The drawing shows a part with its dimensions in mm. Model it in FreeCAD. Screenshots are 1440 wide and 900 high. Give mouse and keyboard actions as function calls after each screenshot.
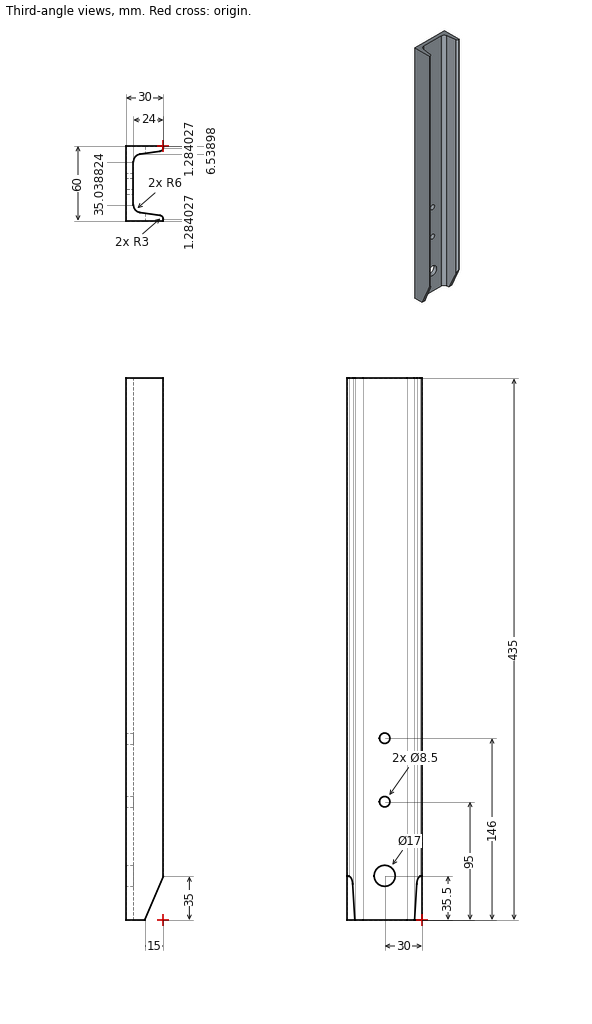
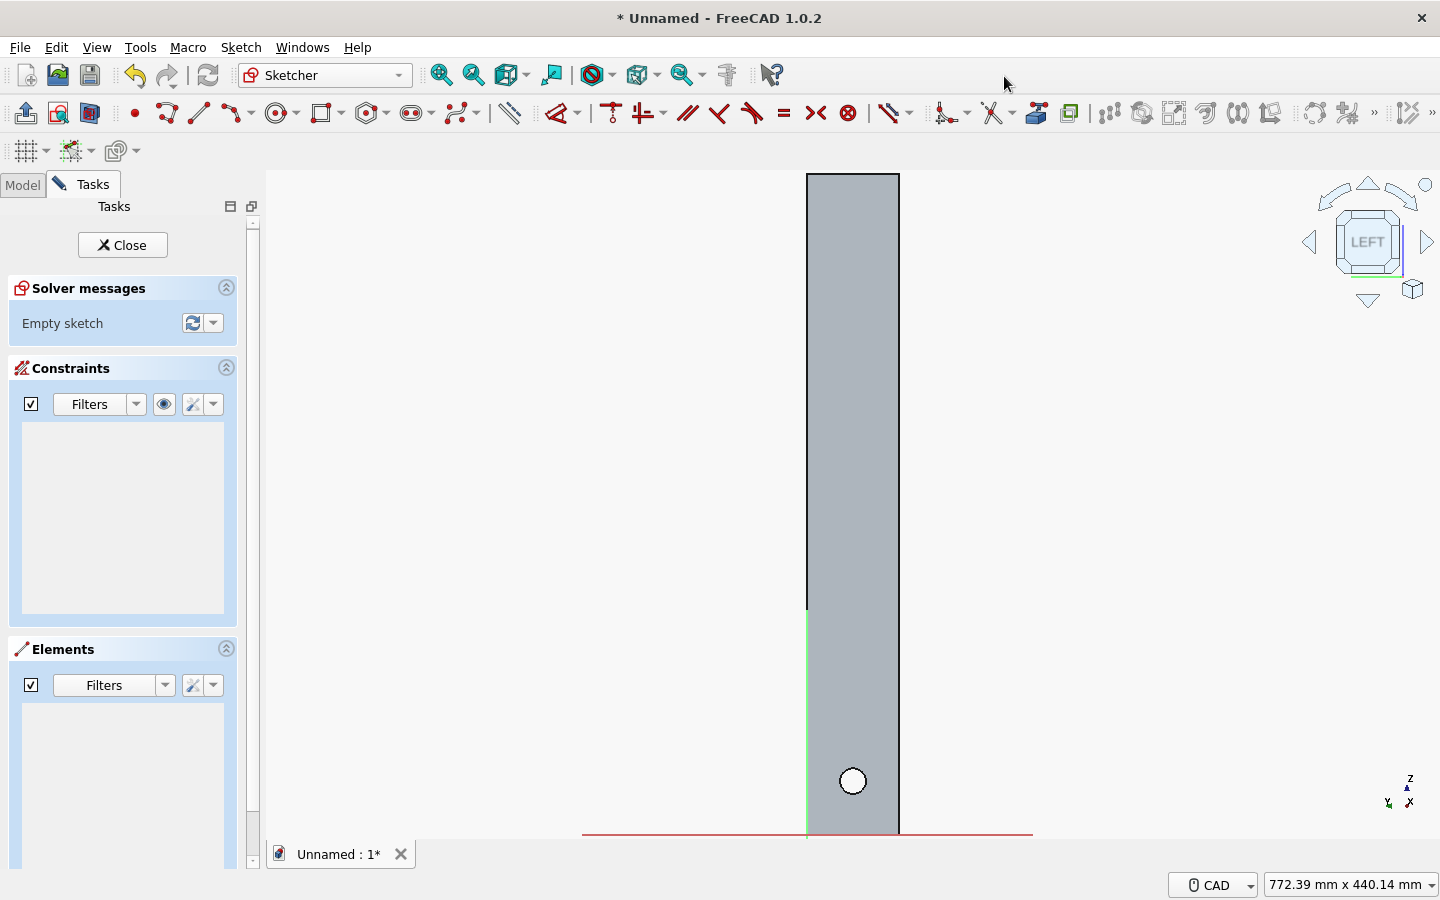
scroll(870, 689, up, 8)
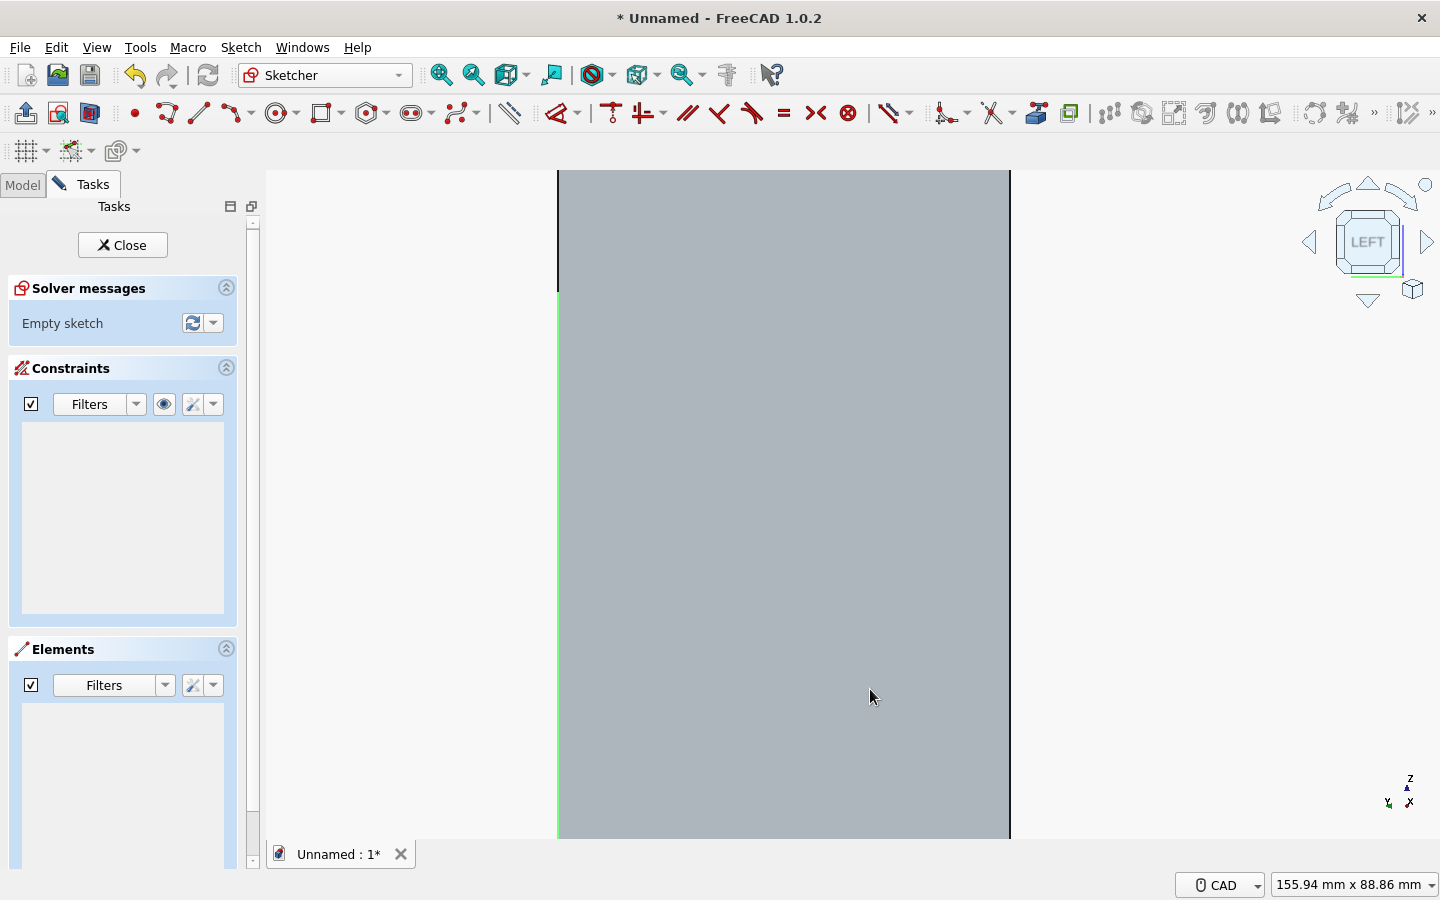
key(g)
key(c)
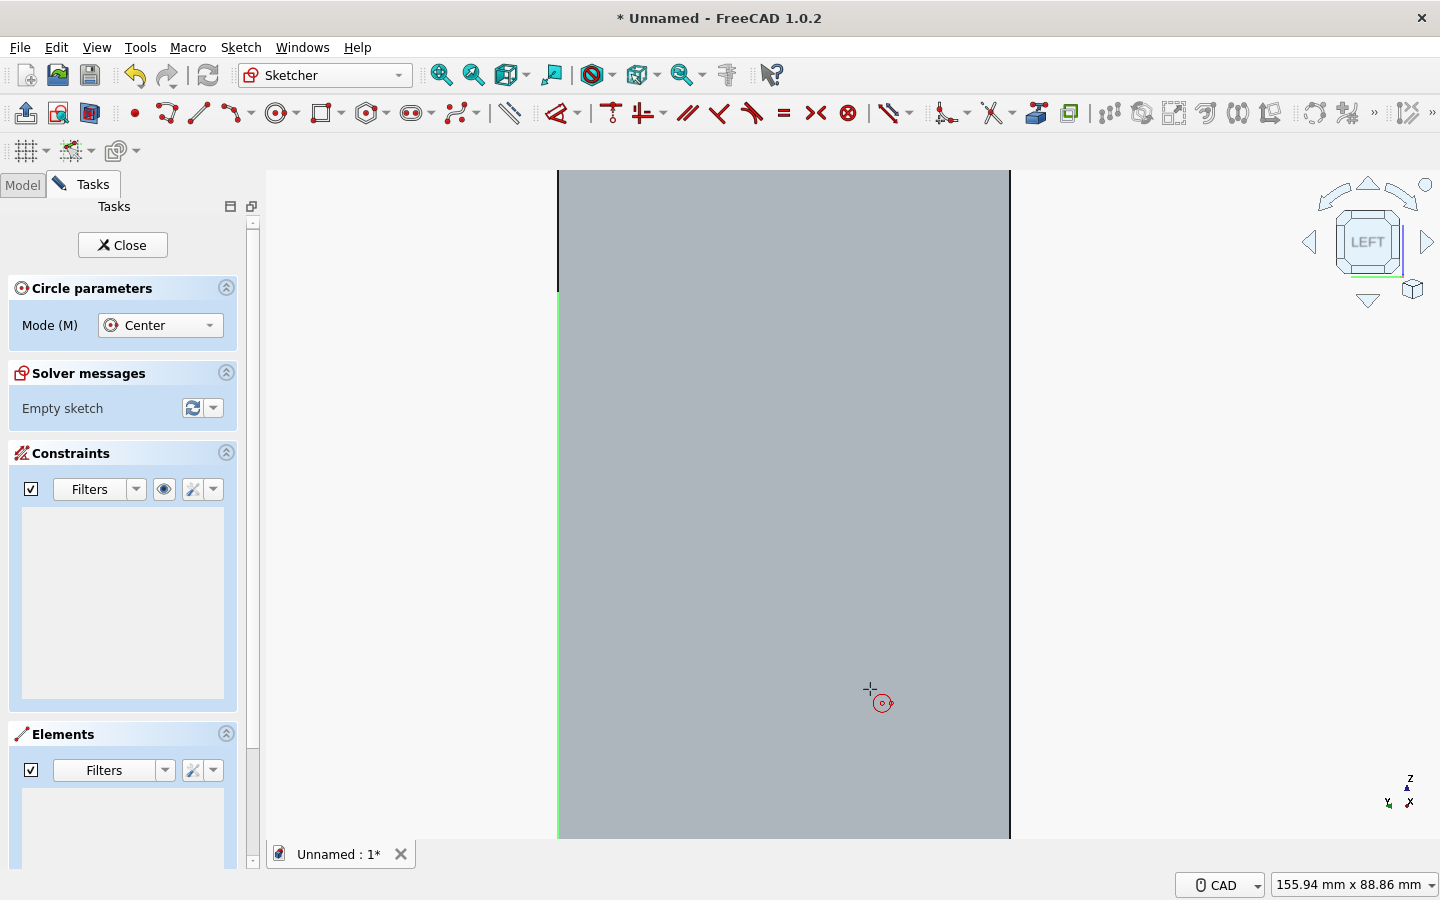
click(784, 694)
move(806, 672)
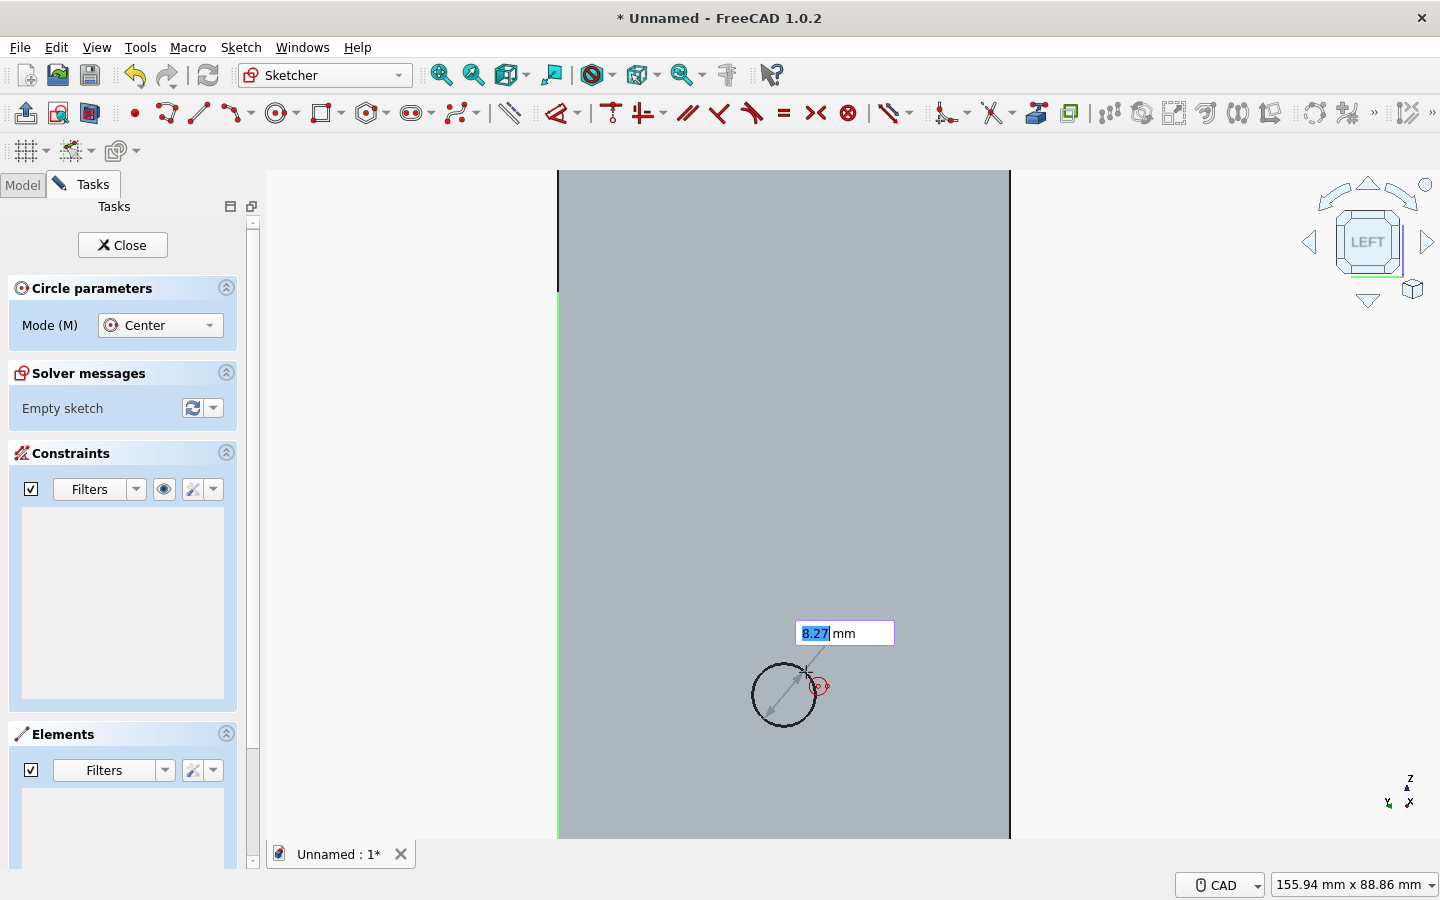
text(8.5)
key(Return)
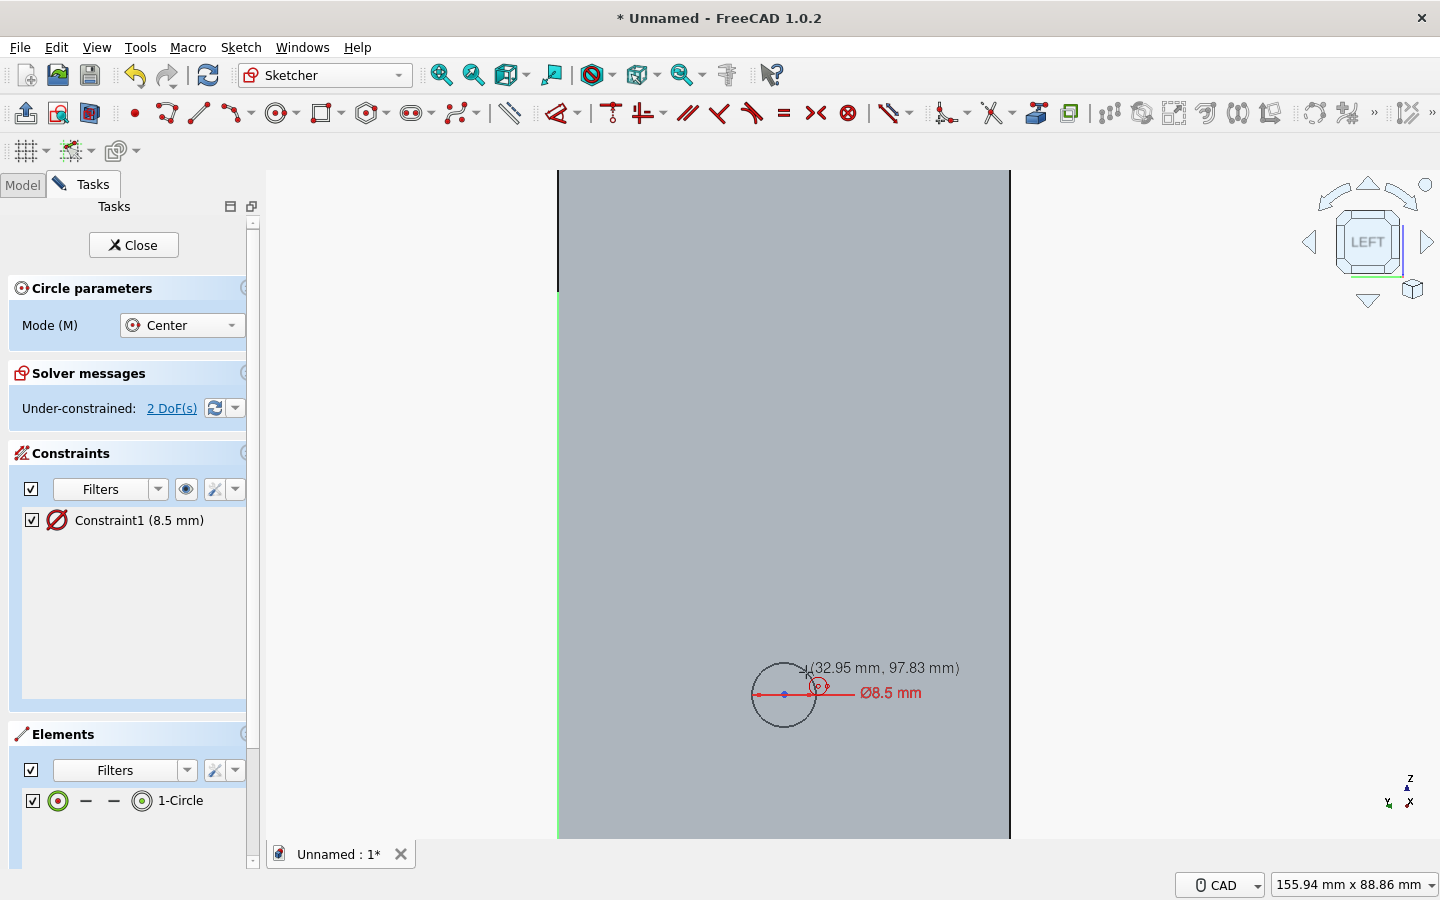
click(784, 310)
move(806, 288)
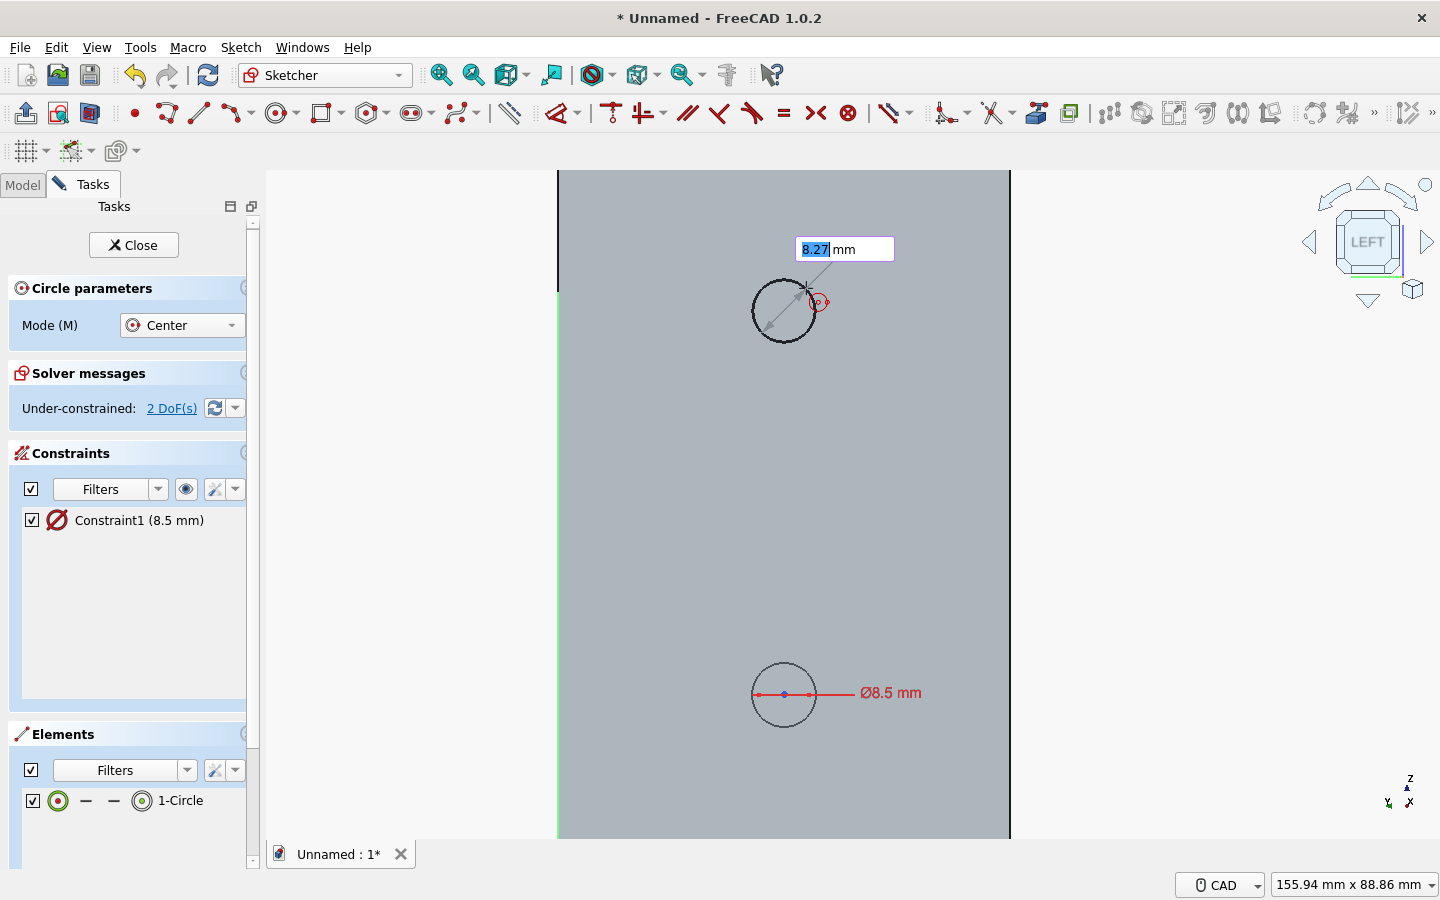
text(8.5)
key(Return)
key(Escape)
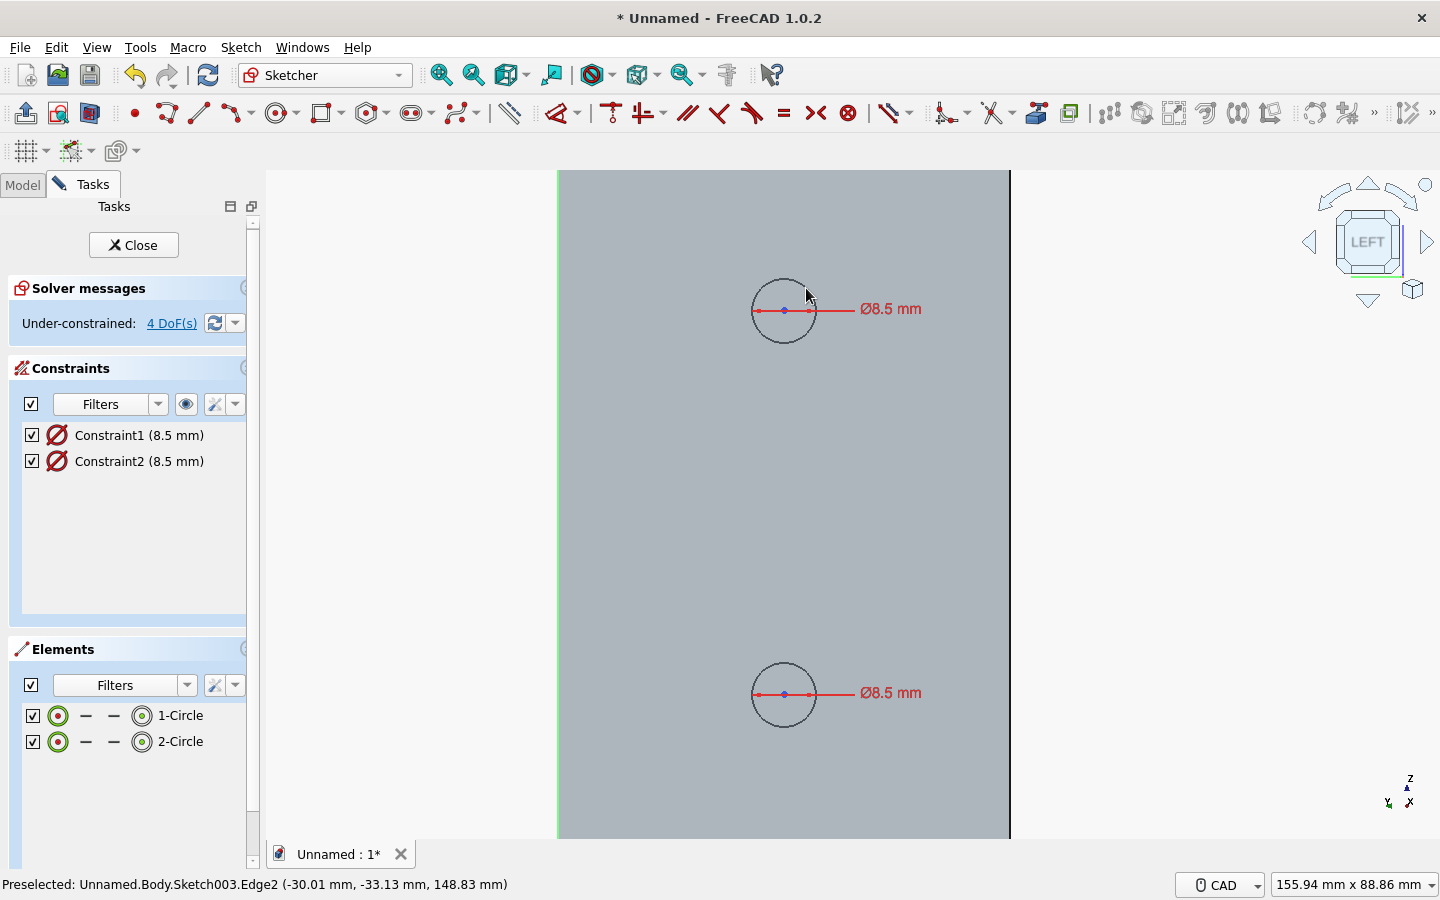
key(d)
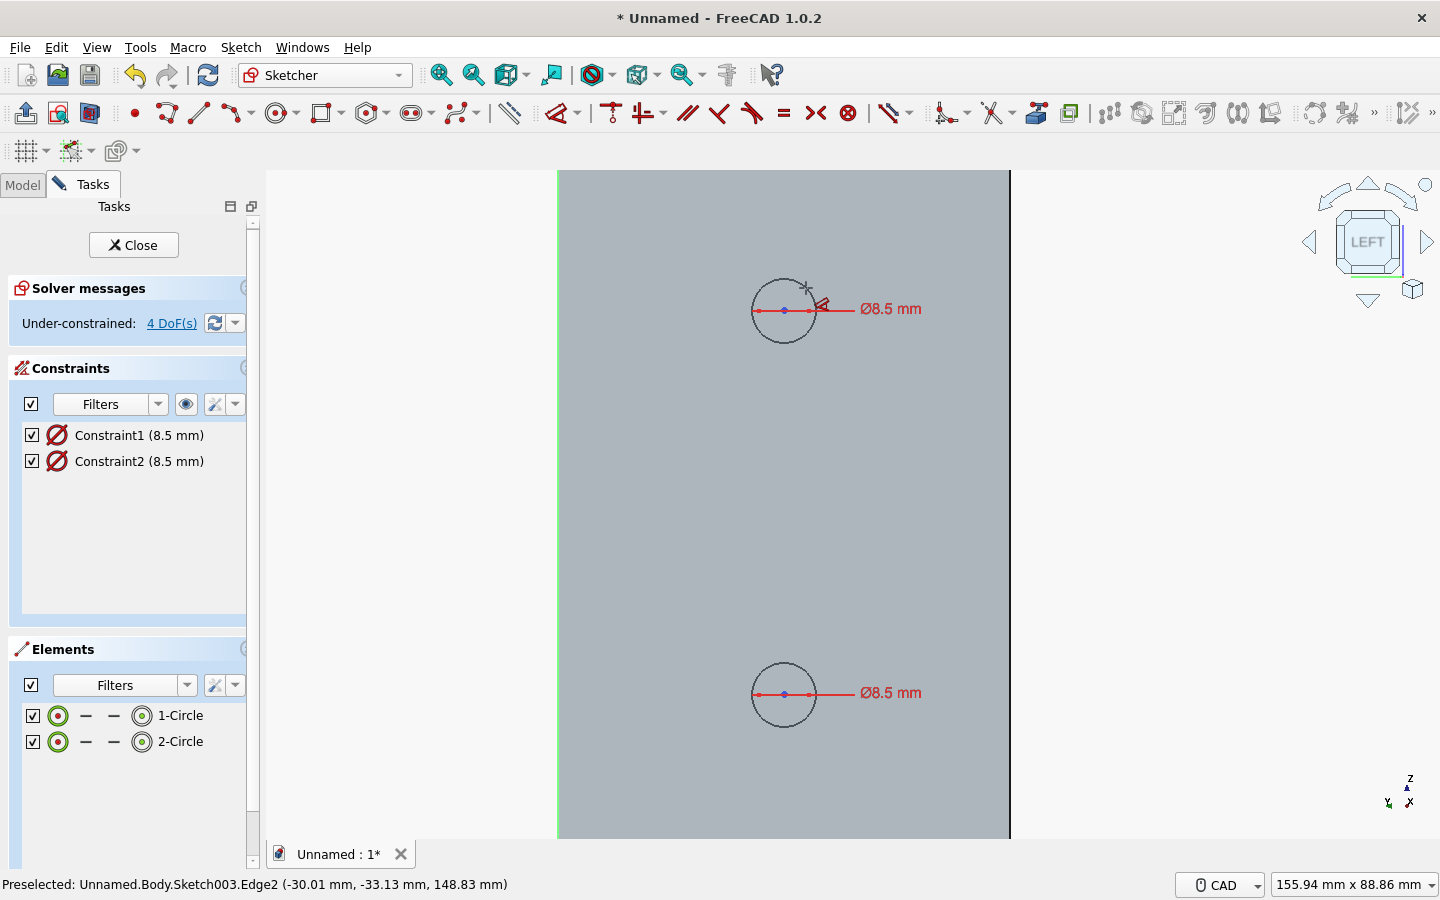
click(784, 695)
click(671, 661)